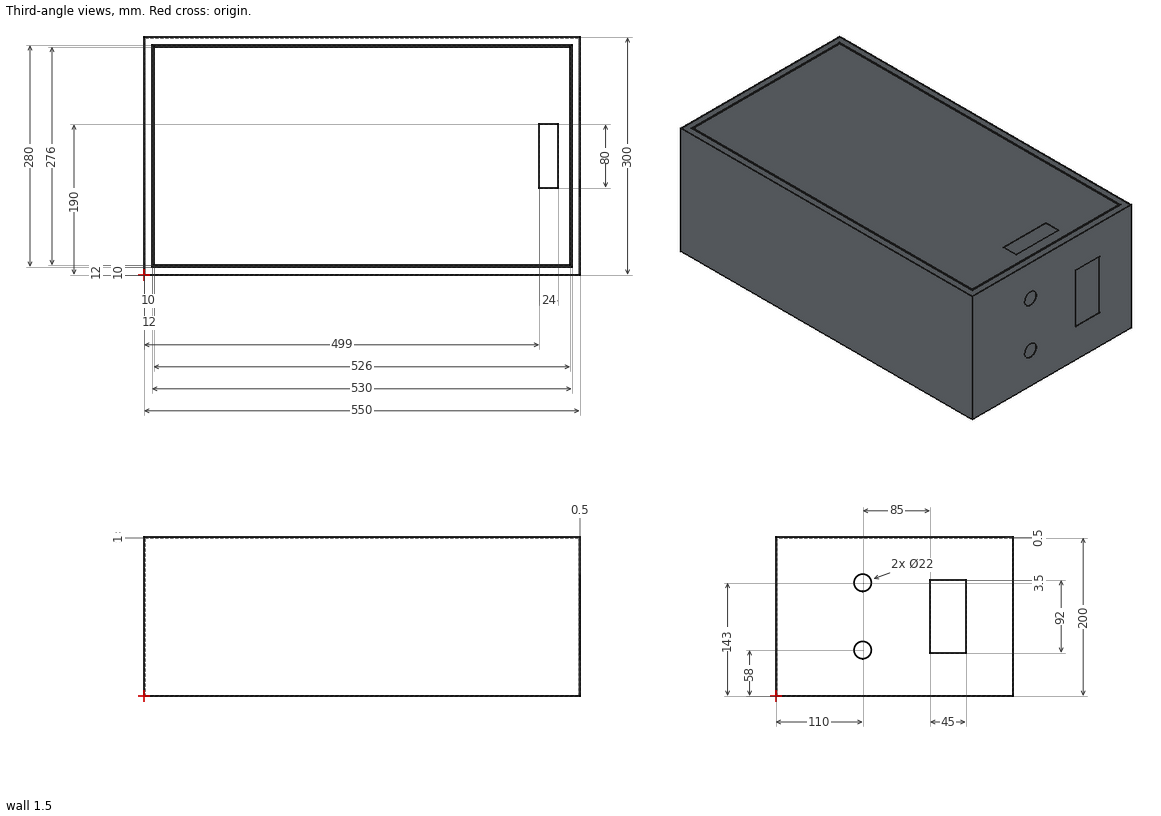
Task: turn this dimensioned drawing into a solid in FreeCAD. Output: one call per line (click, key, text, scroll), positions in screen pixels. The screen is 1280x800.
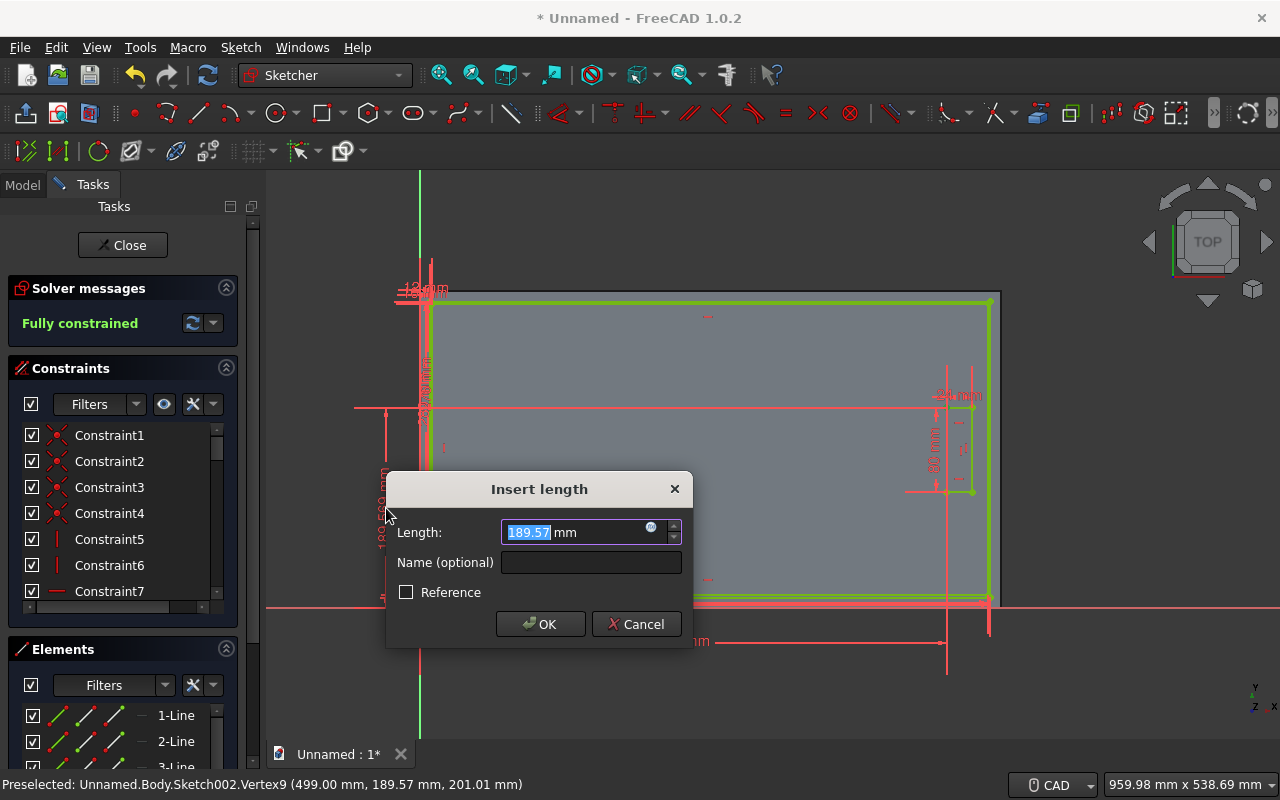
text(190)
key(Return)
key(Escape)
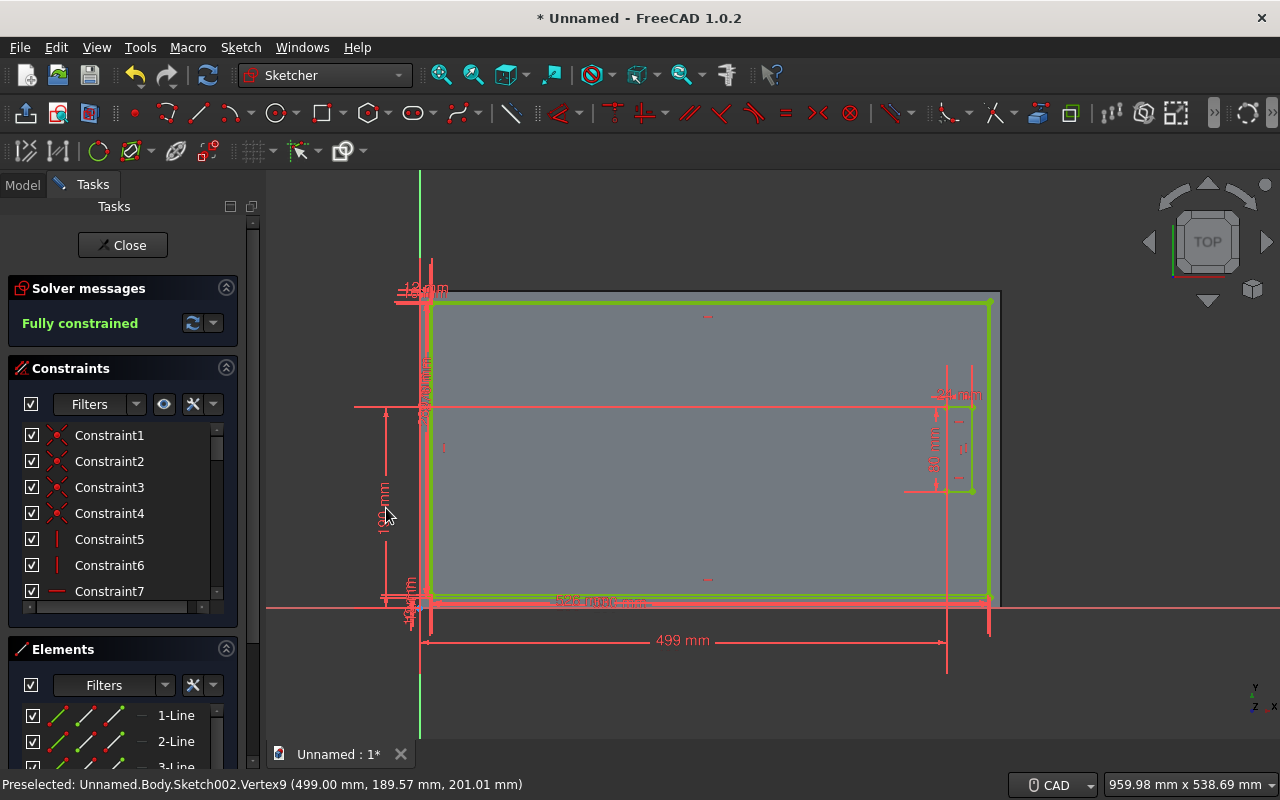
click(123, 245)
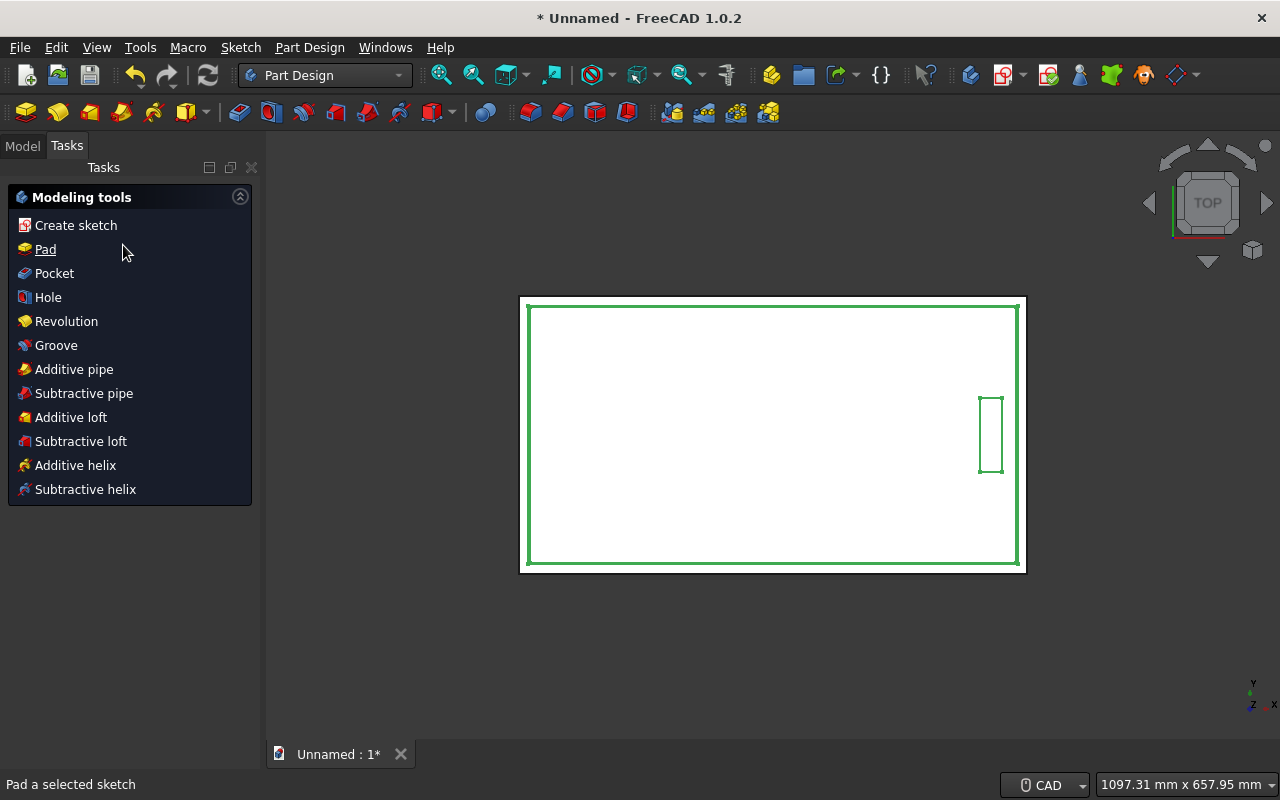
click(240, 112)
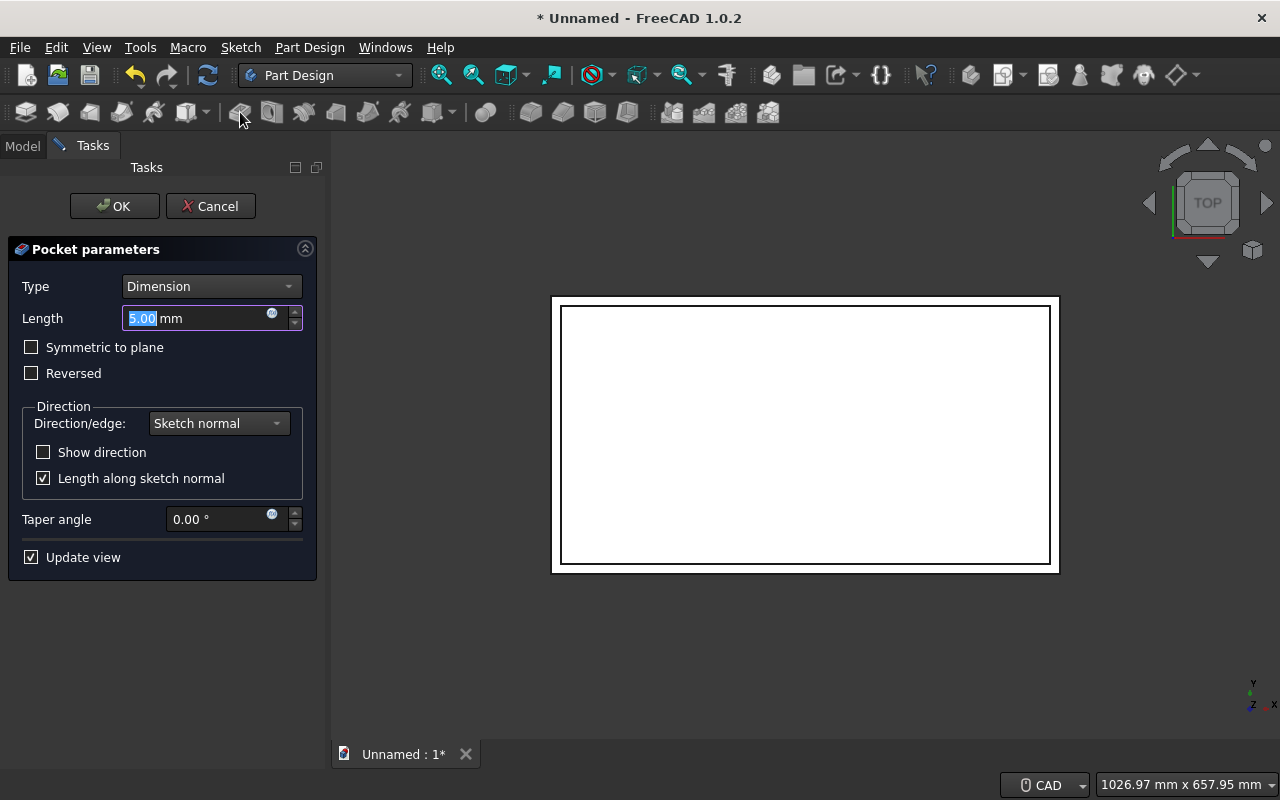
text(0.5)
key(Tab)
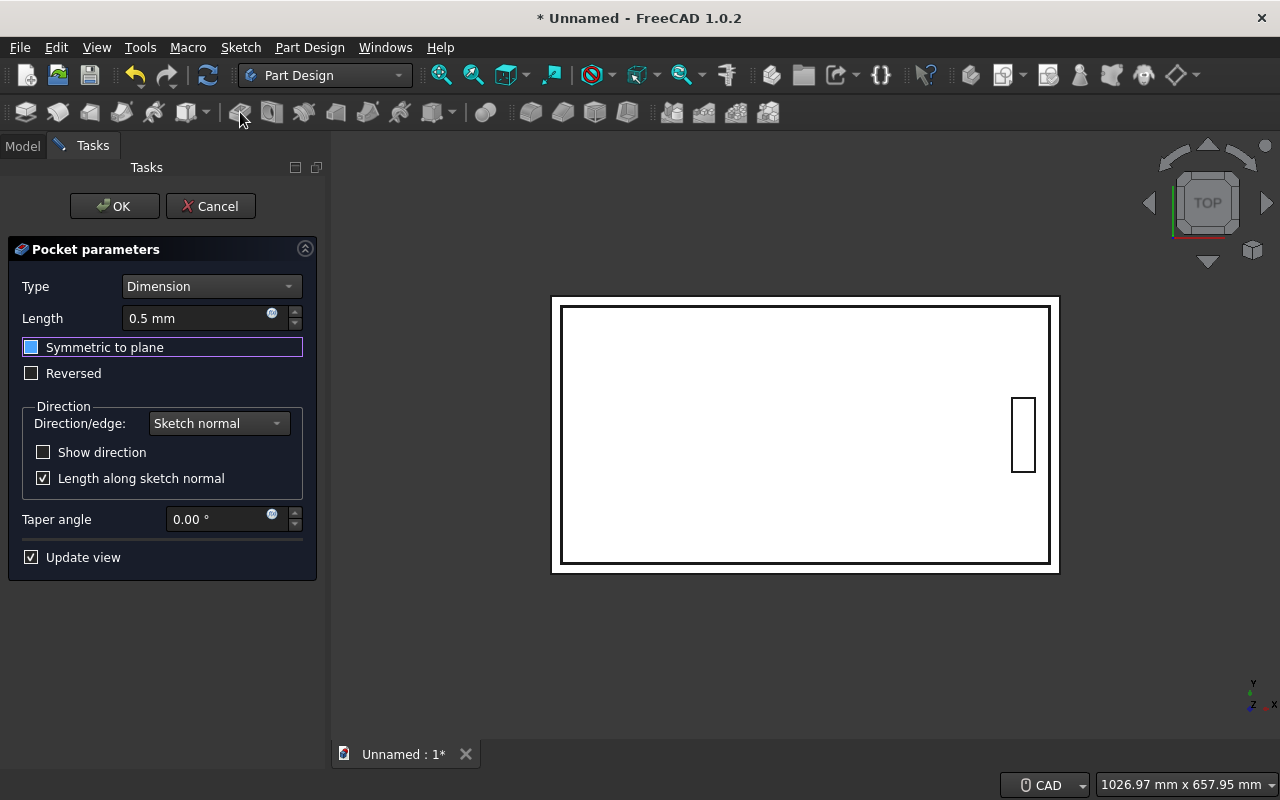
click(115, 206)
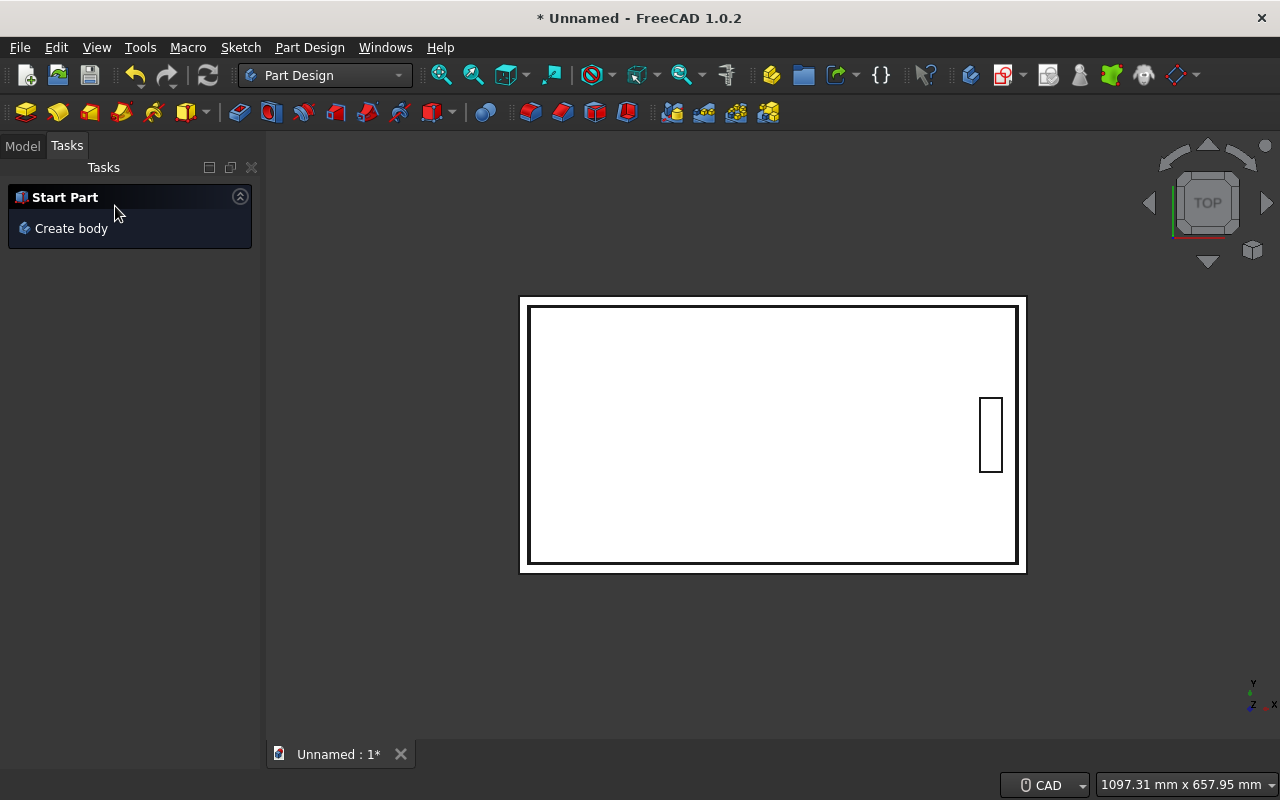
key(0)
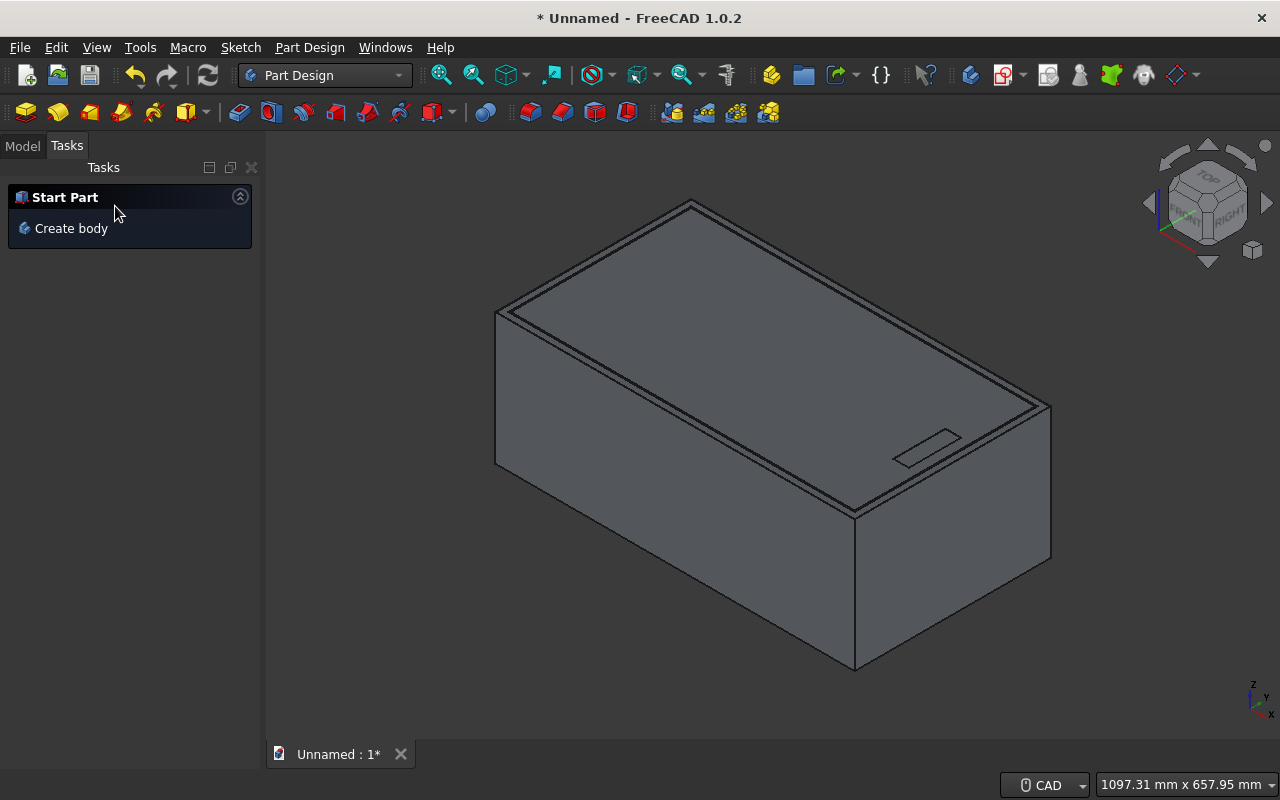
click(981, 522)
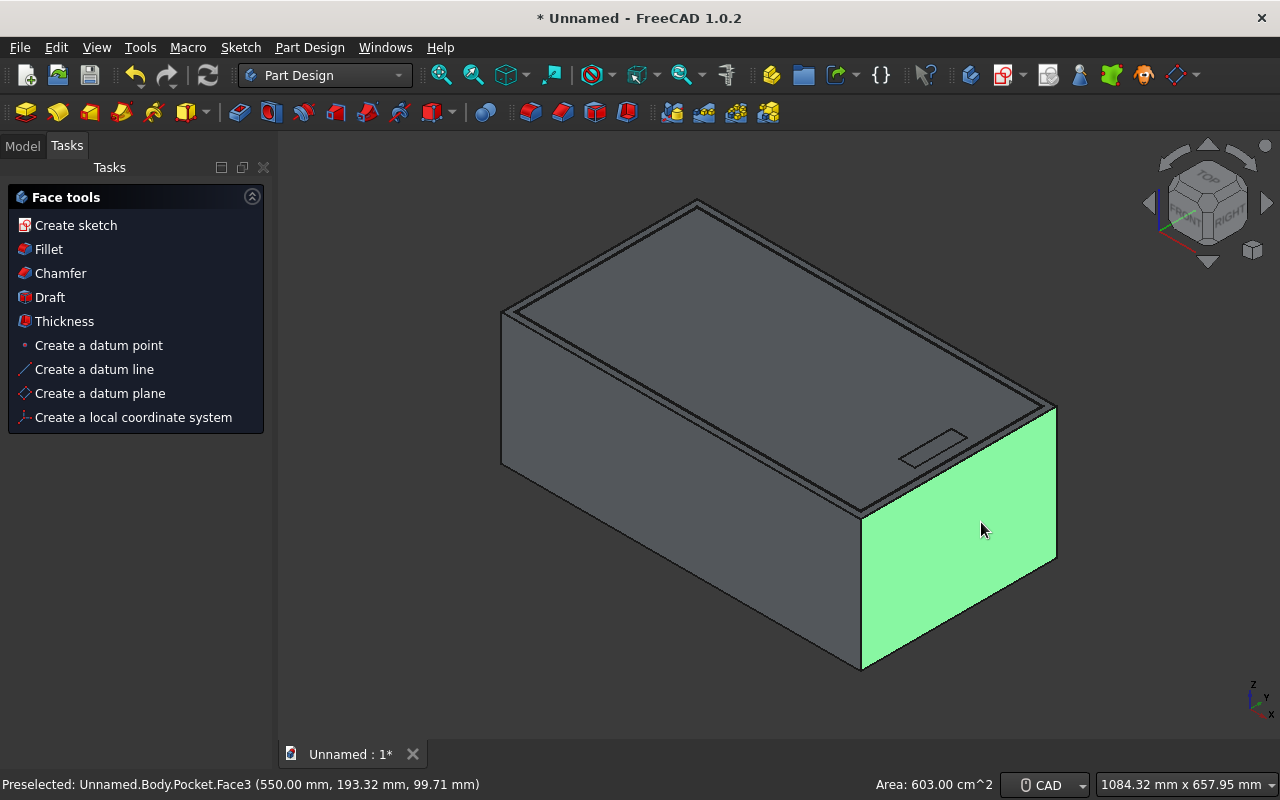
click(1004, 76)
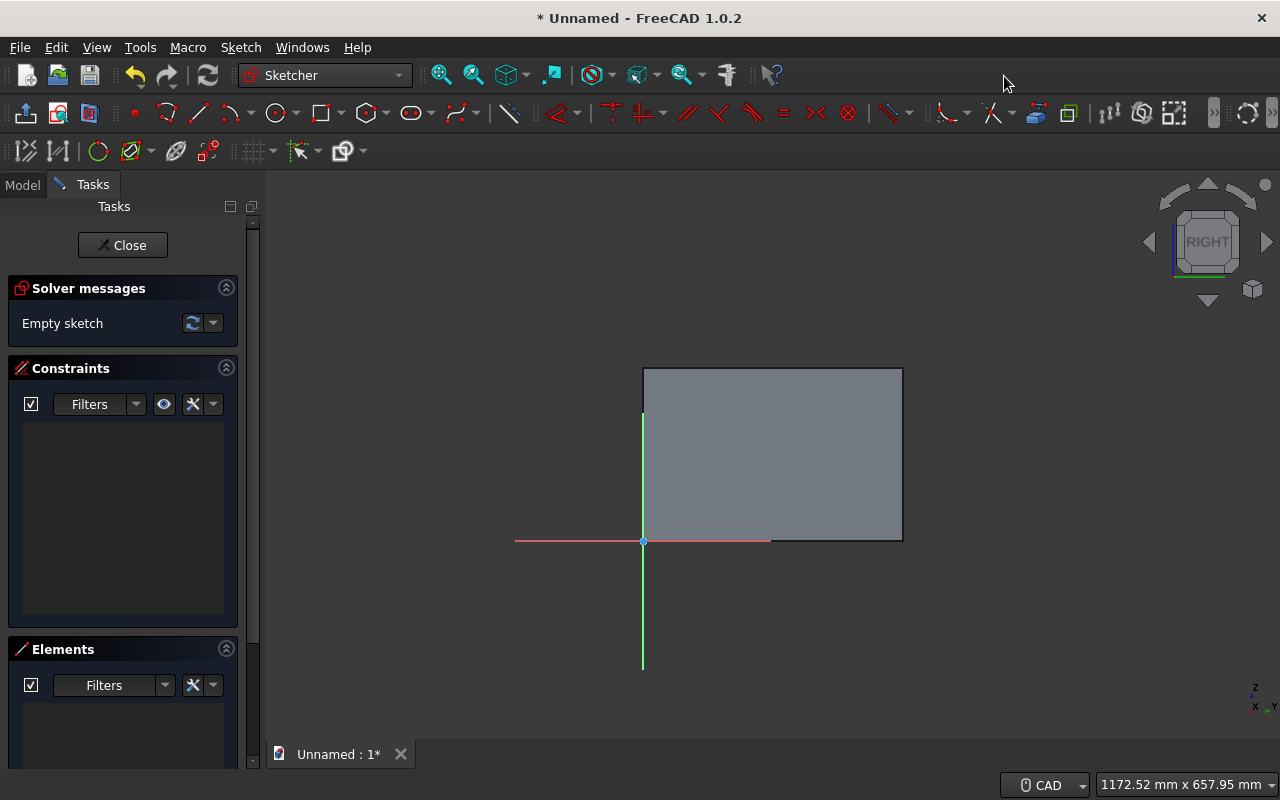
scroll(772, 487, up, 5)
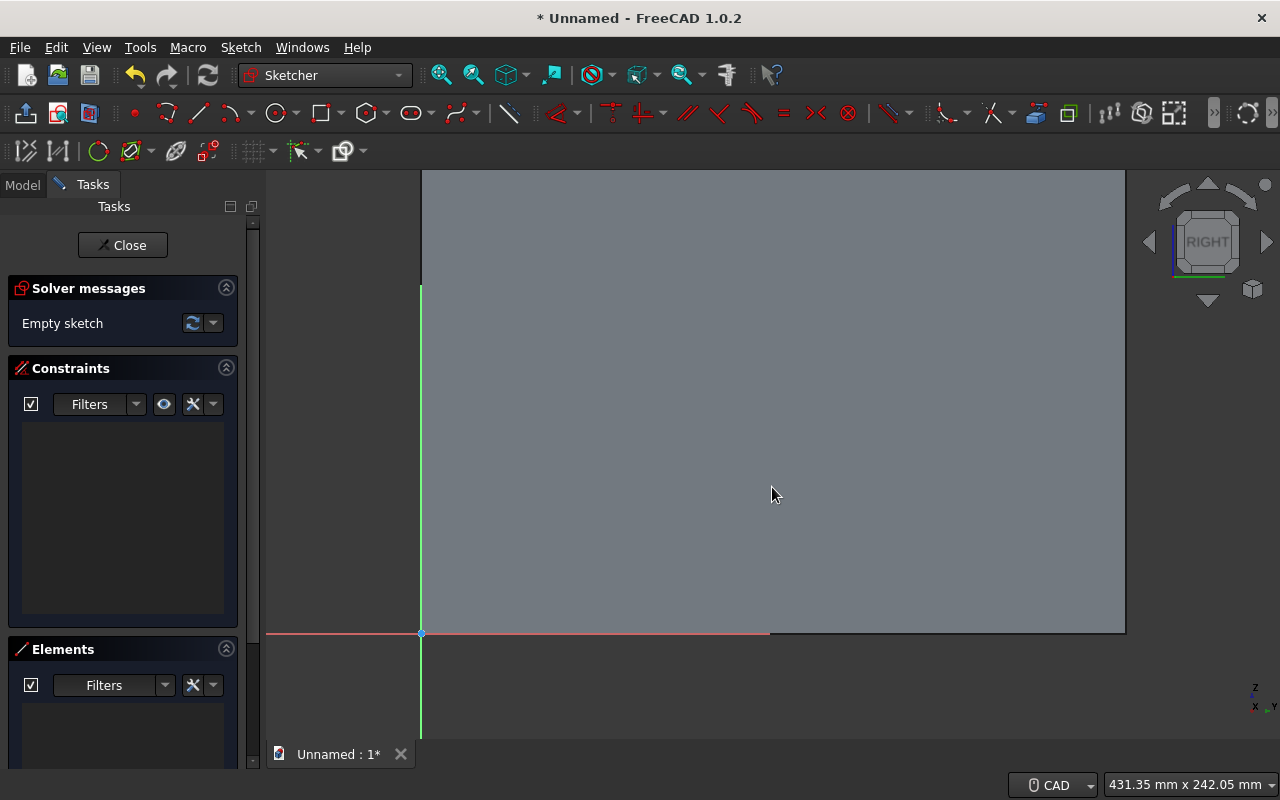
click(322, 114)